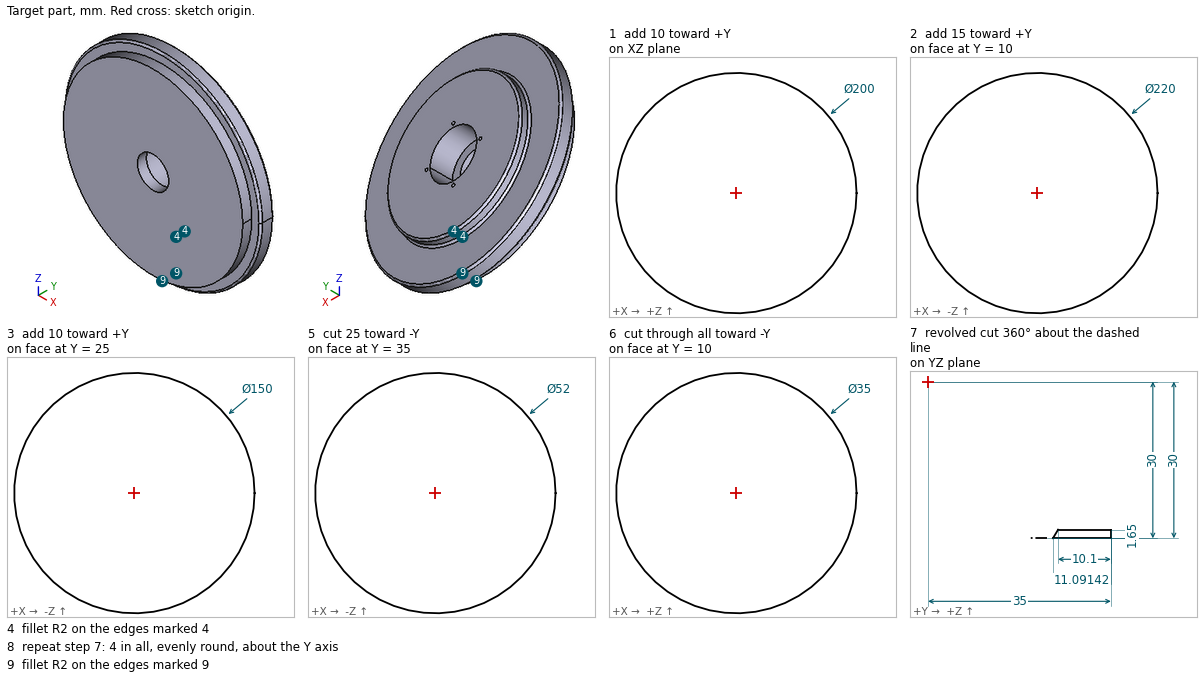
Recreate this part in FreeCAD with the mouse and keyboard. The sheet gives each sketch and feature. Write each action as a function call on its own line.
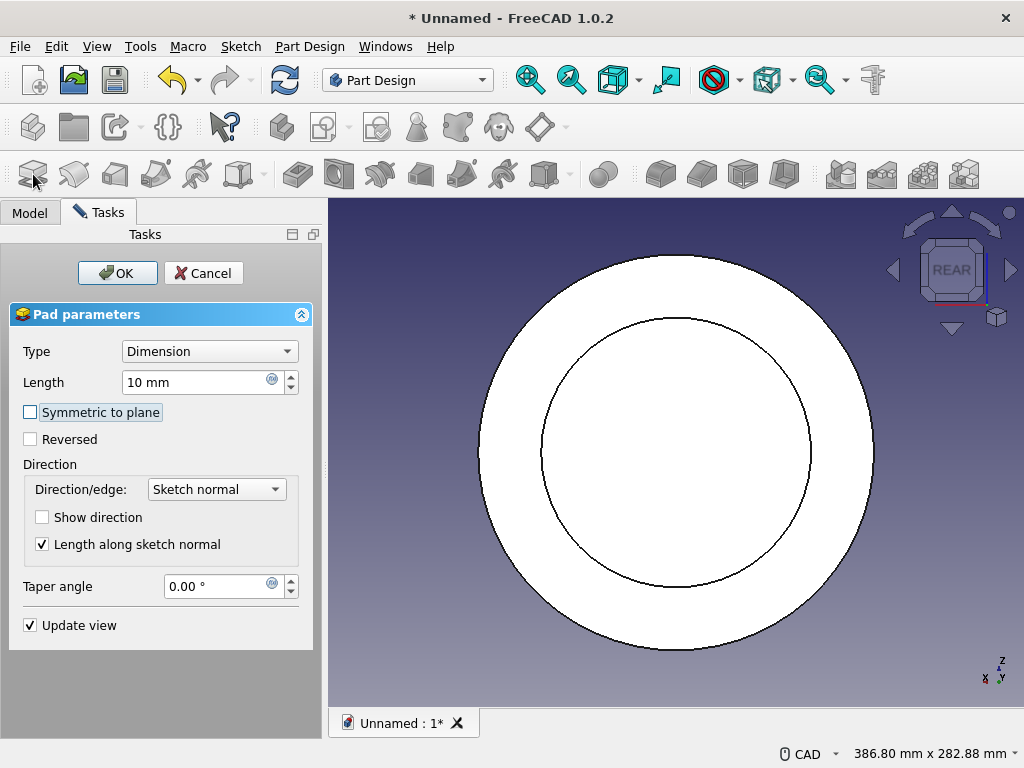
click(118, 273)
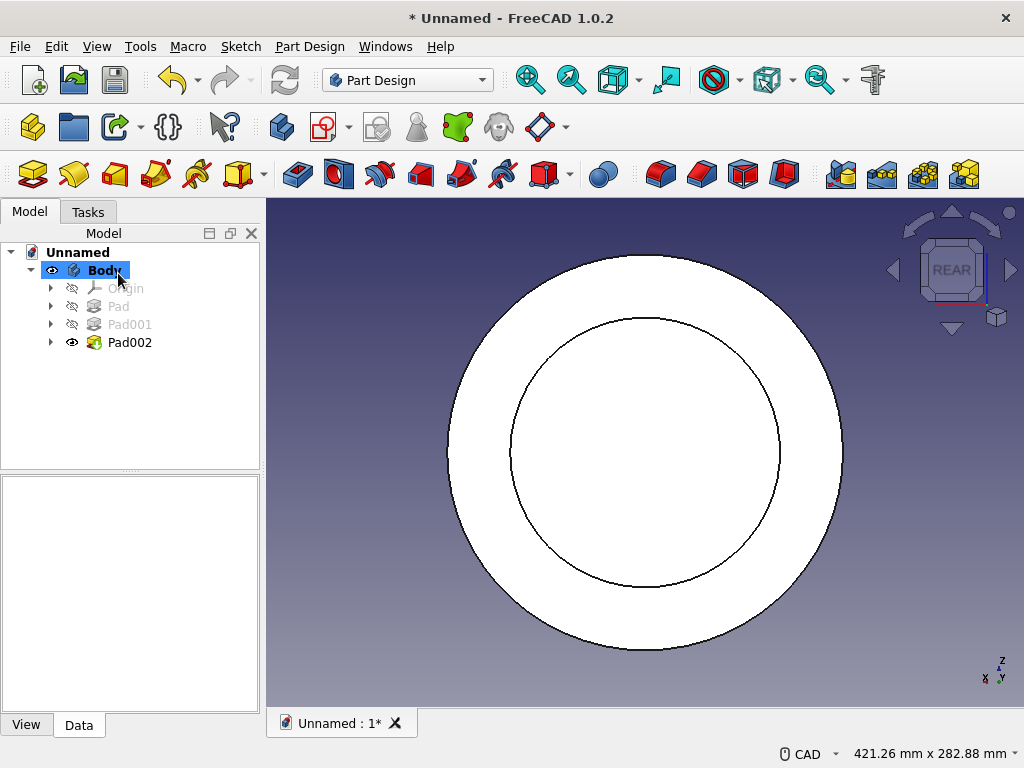
click(780, 452)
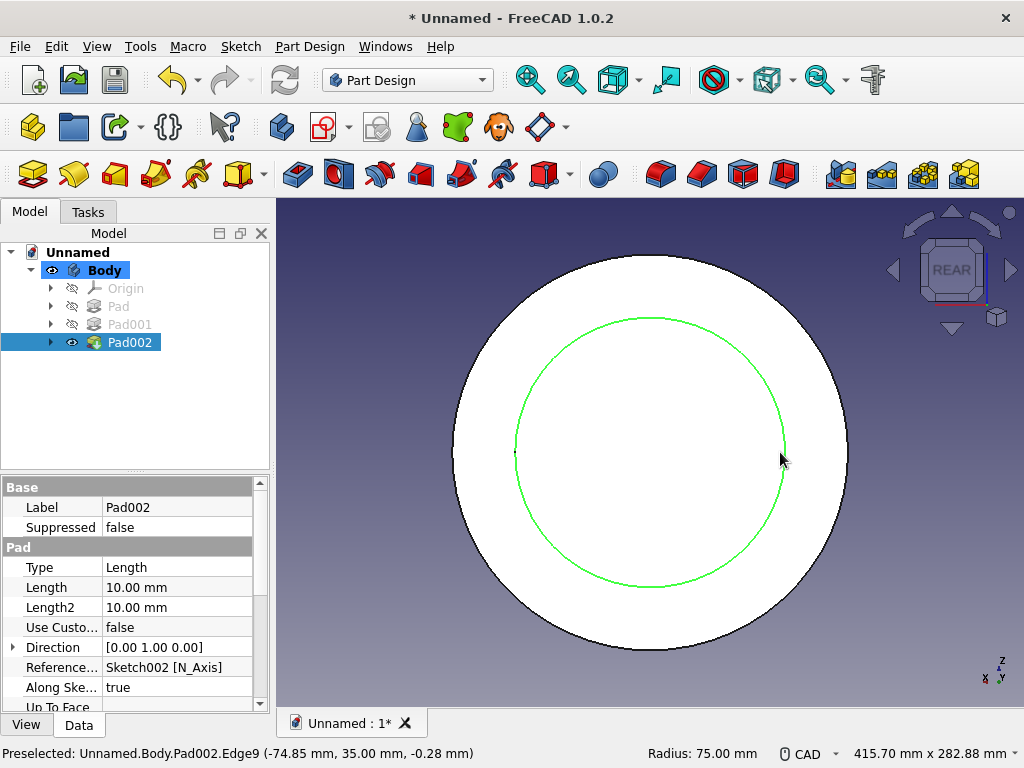
key(0)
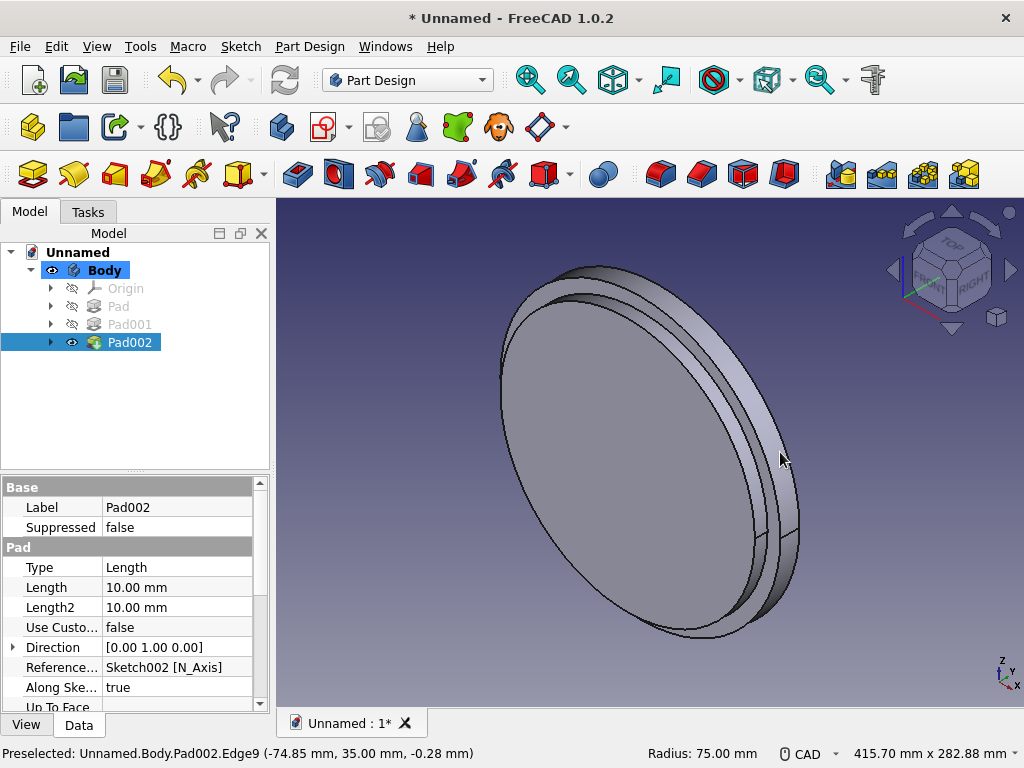
click(531, 80)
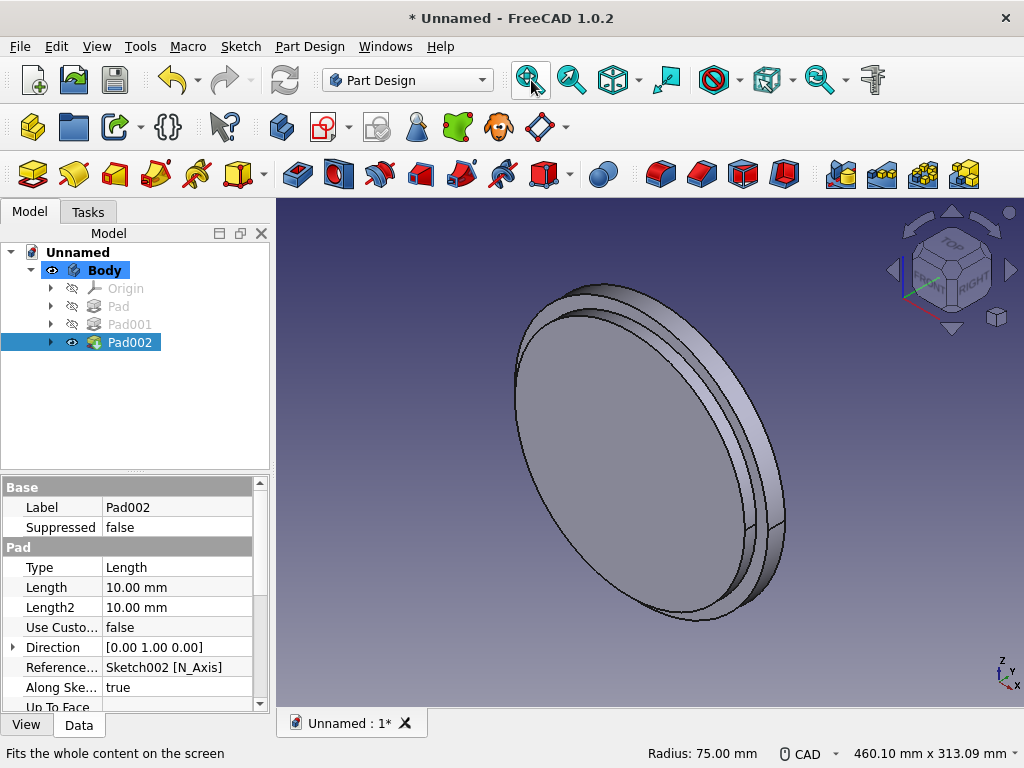
key(2)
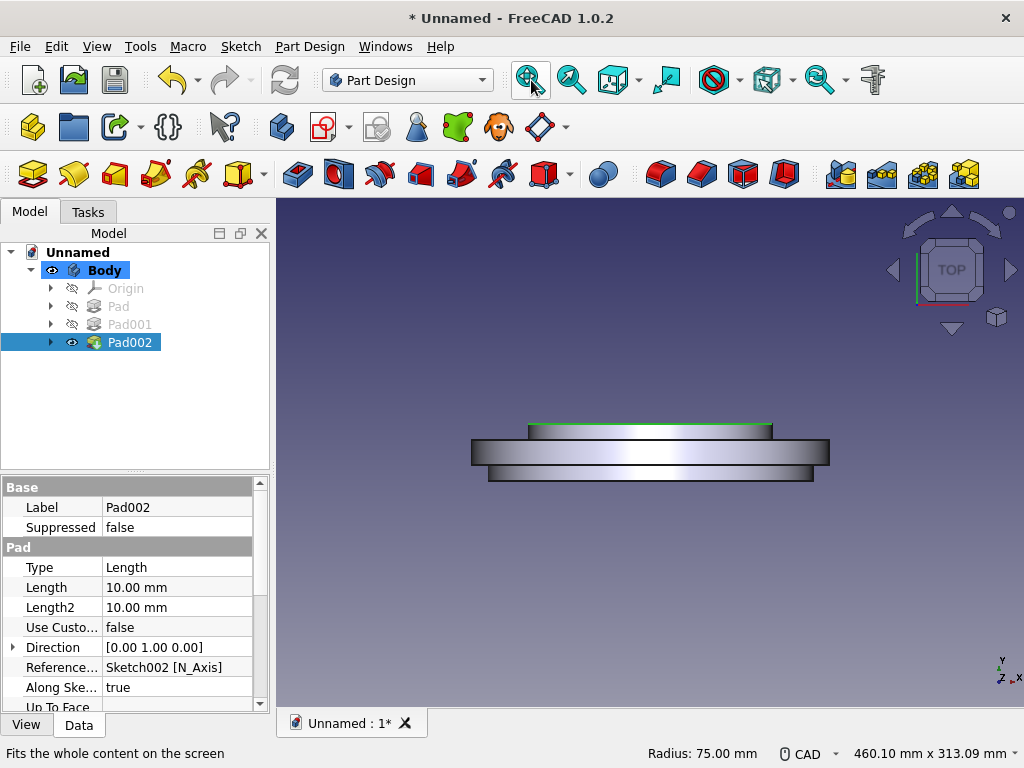
key(1)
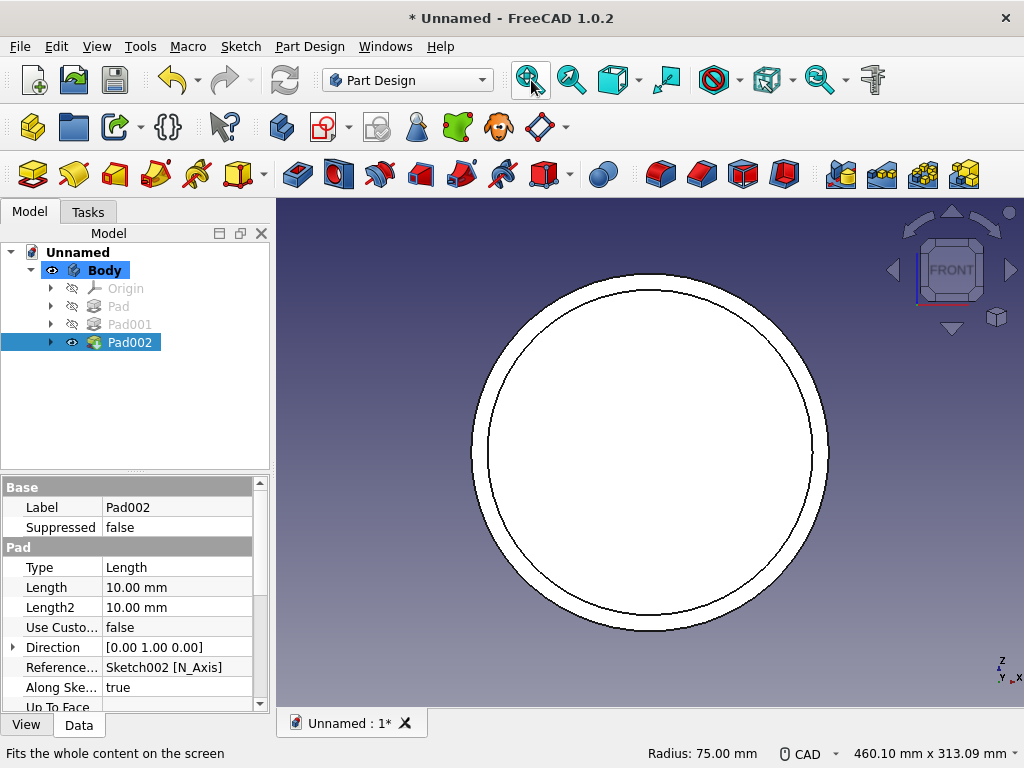
key(3)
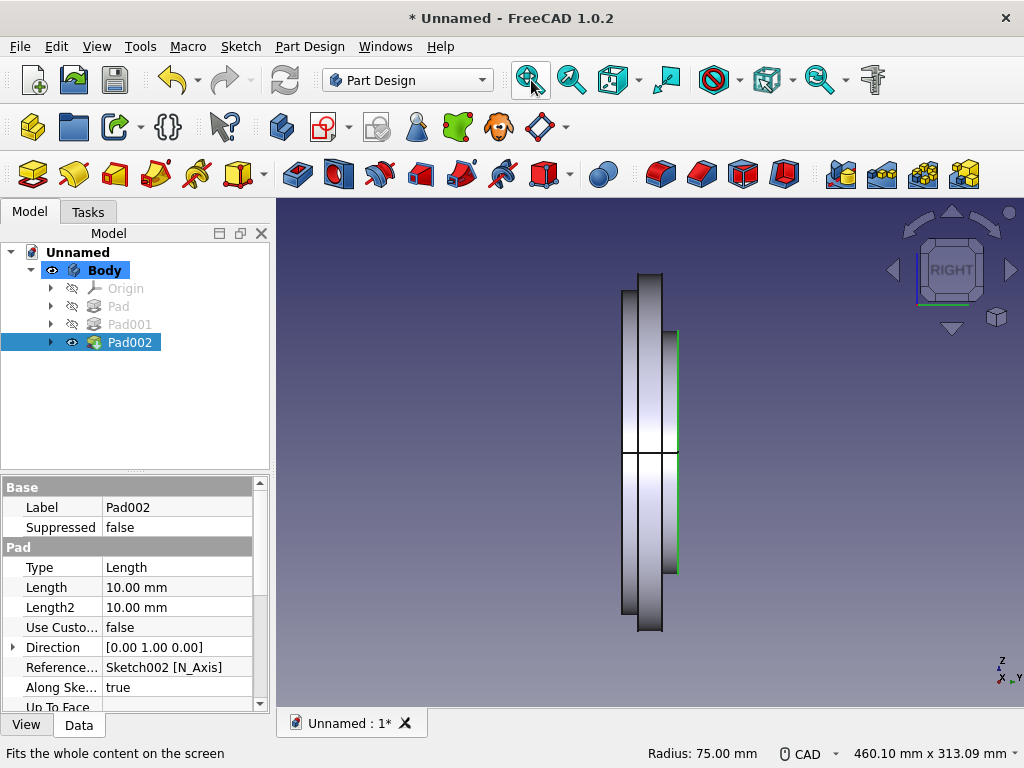
key(5)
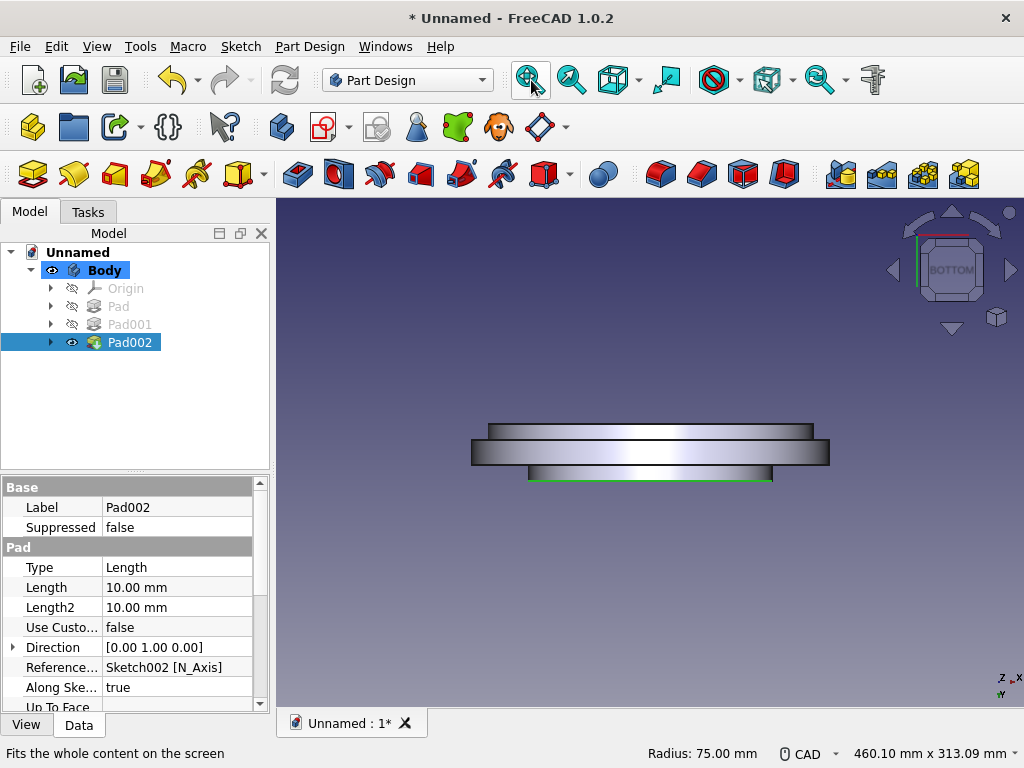
key(4)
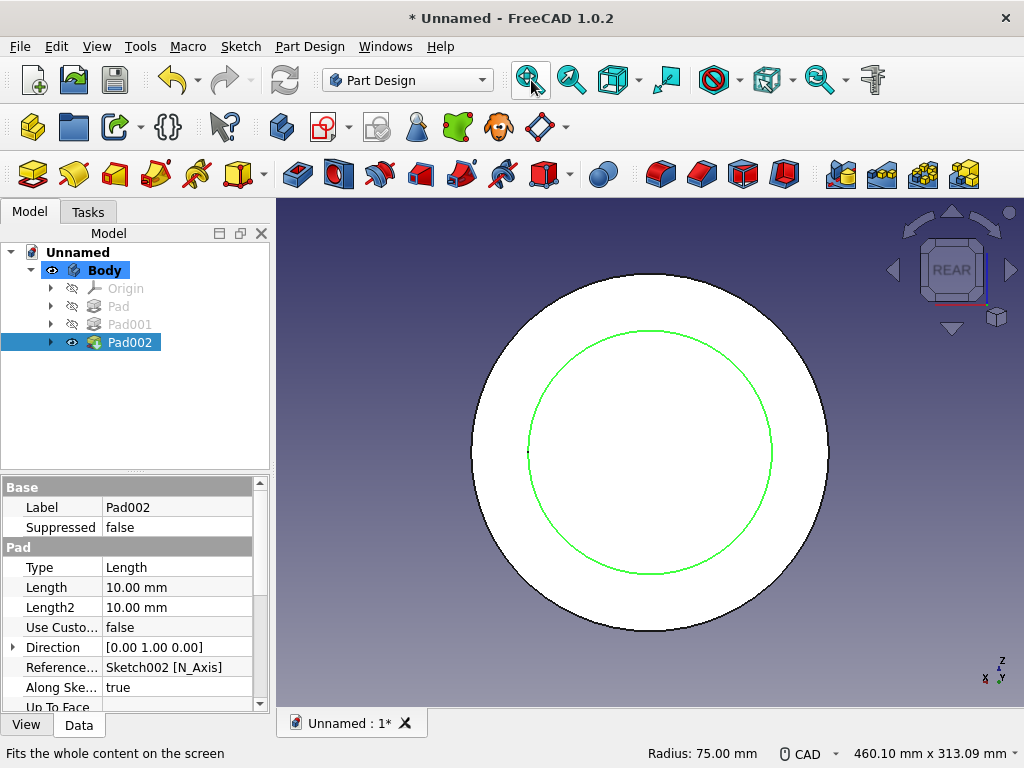
key(6)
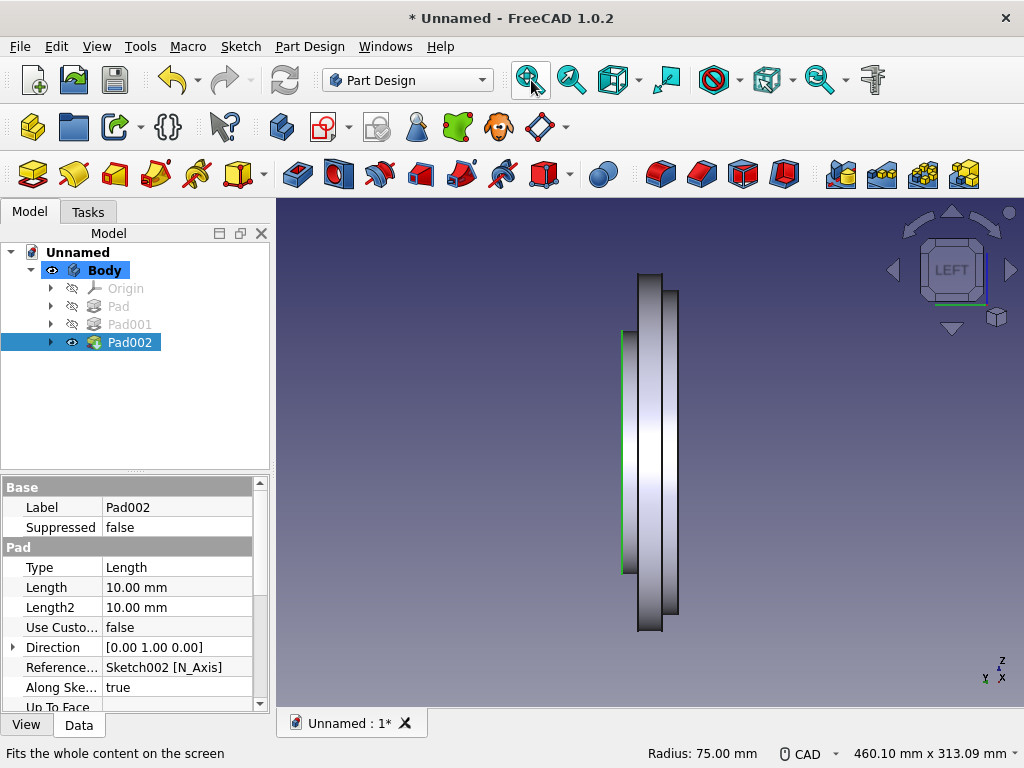
key(v)
key(3)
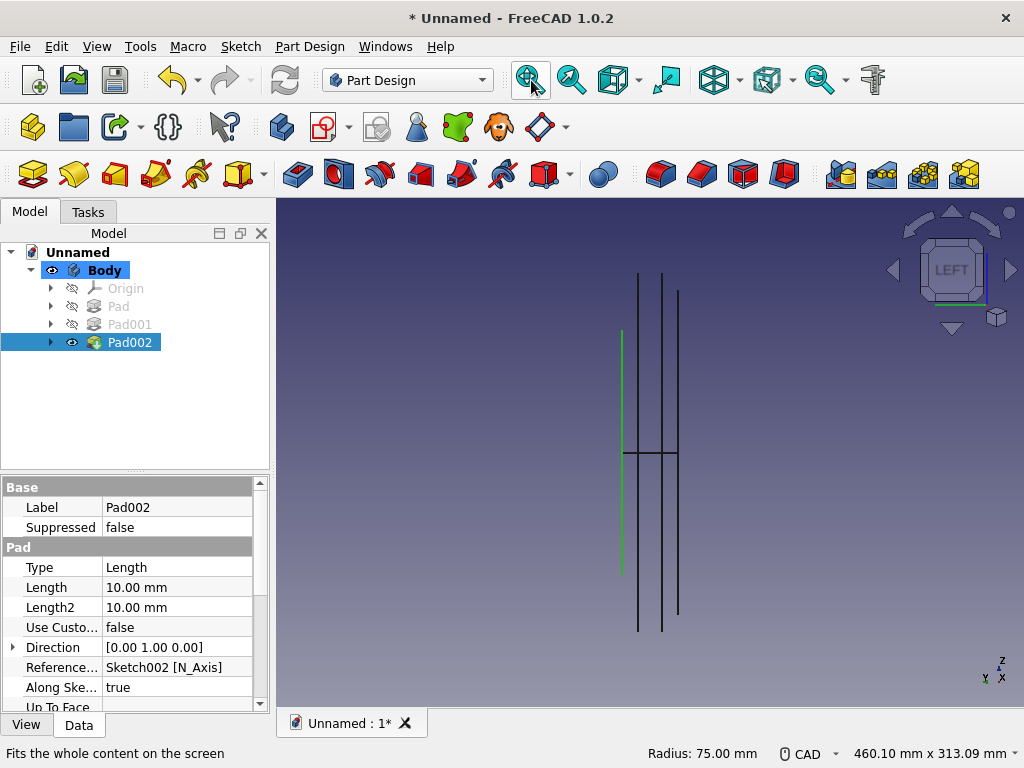
key(0)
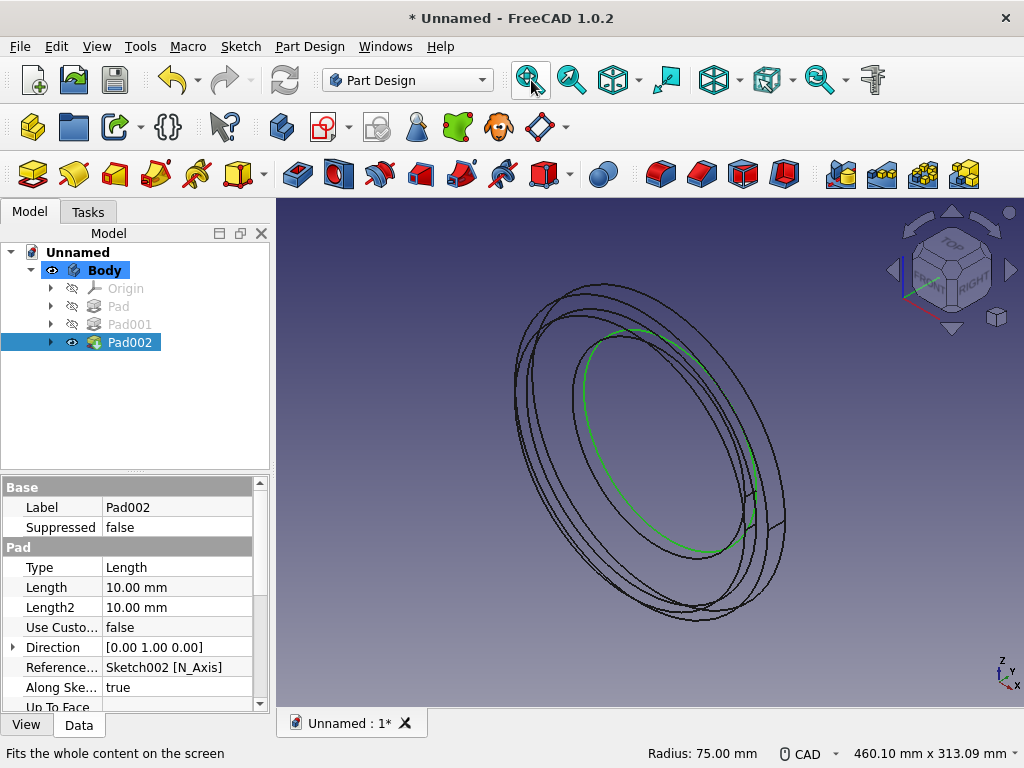
click(572, 397, ctrl)